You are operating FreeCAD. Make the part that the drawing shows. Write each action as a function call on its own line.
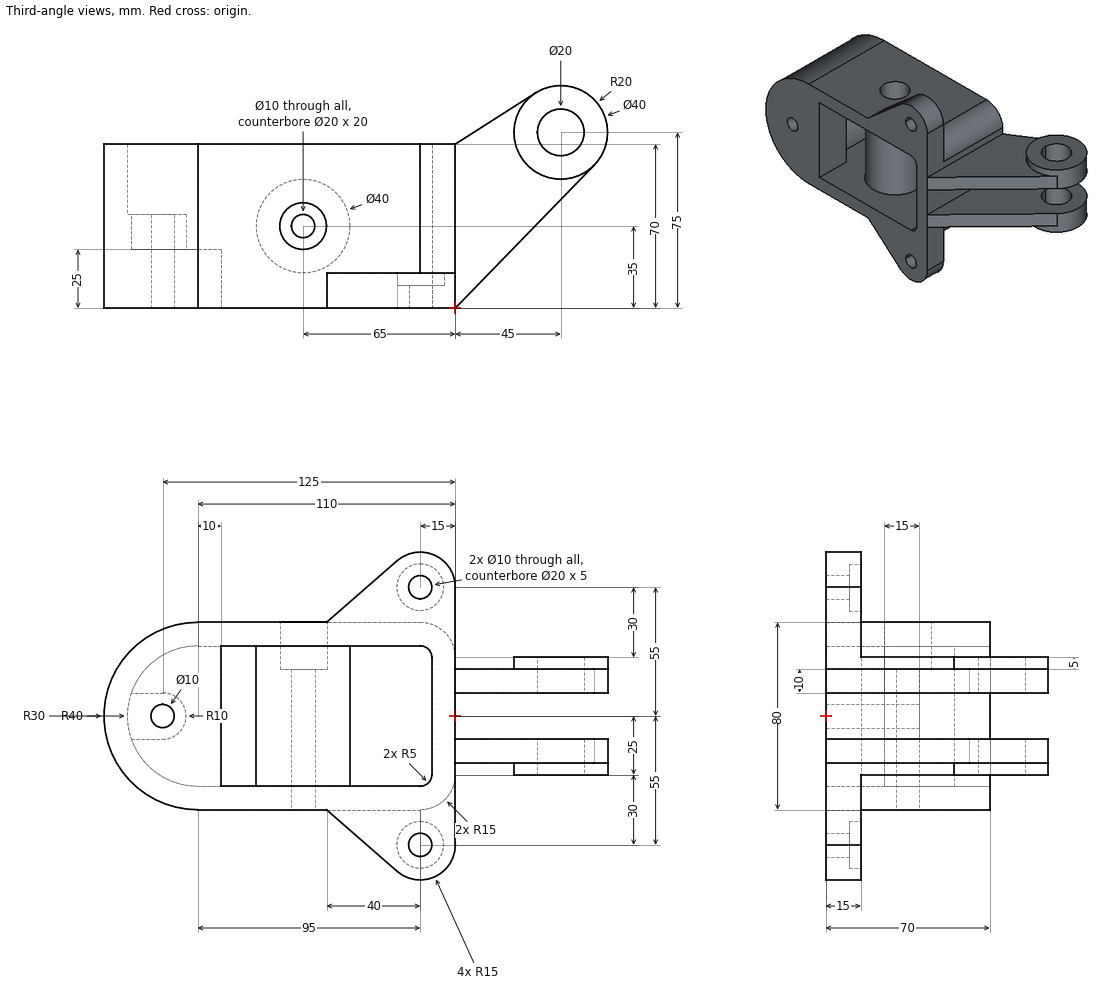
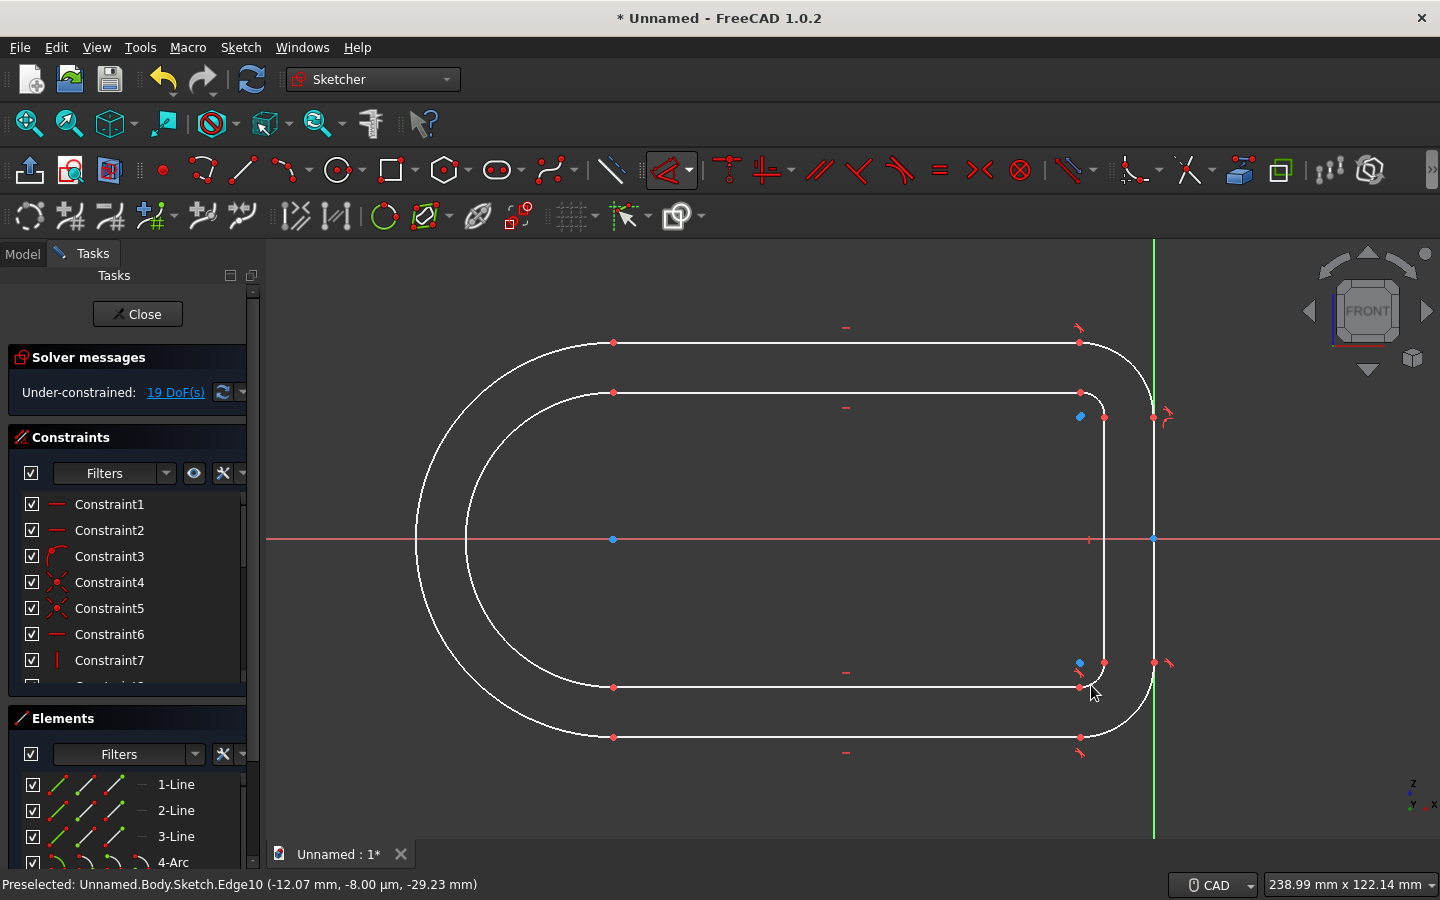
click(754, 687)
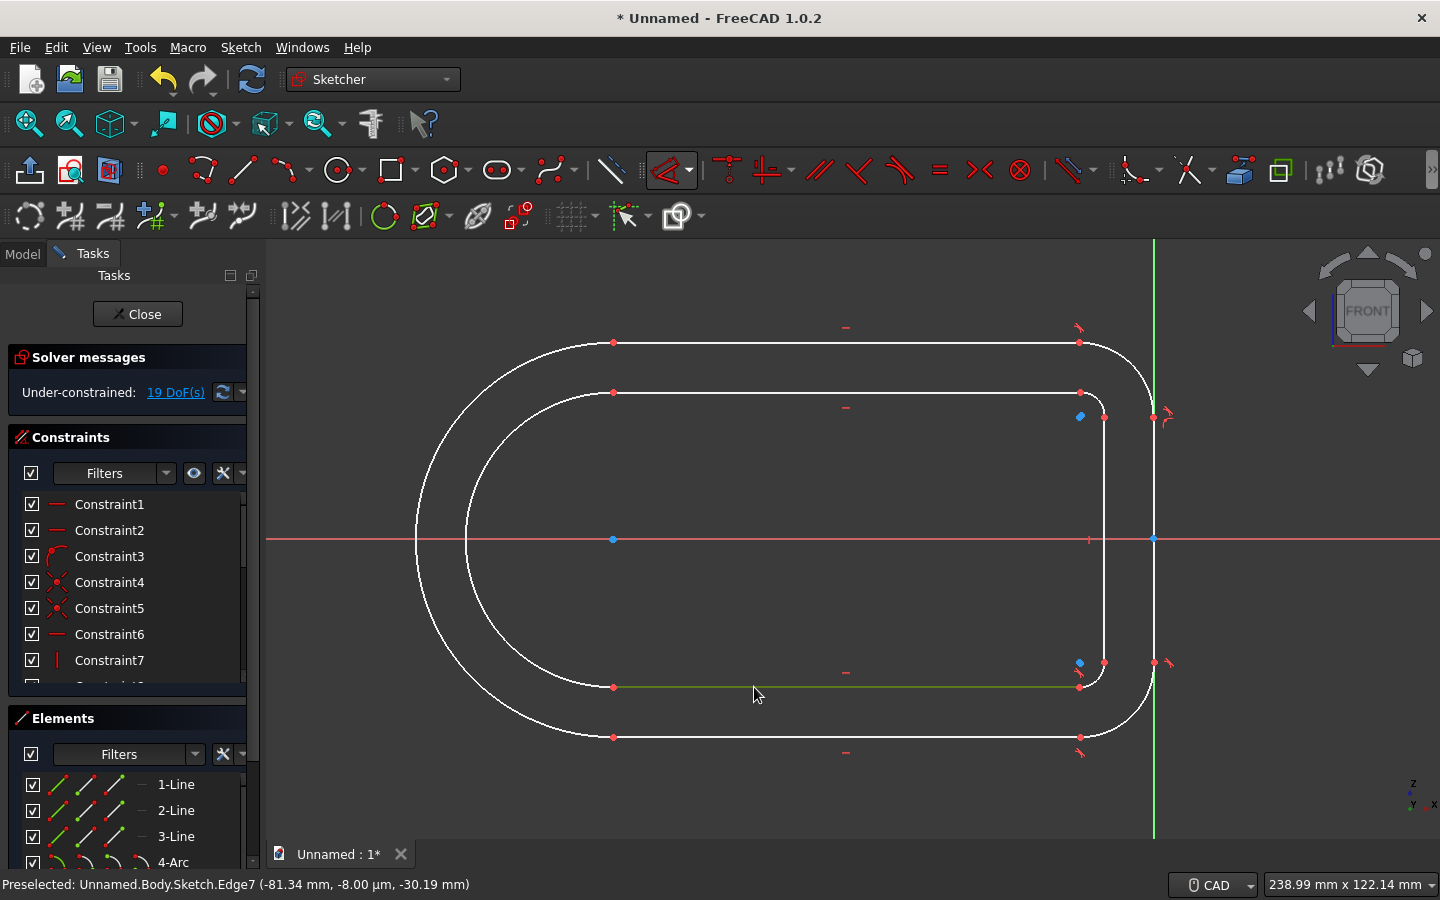
click(494, 453)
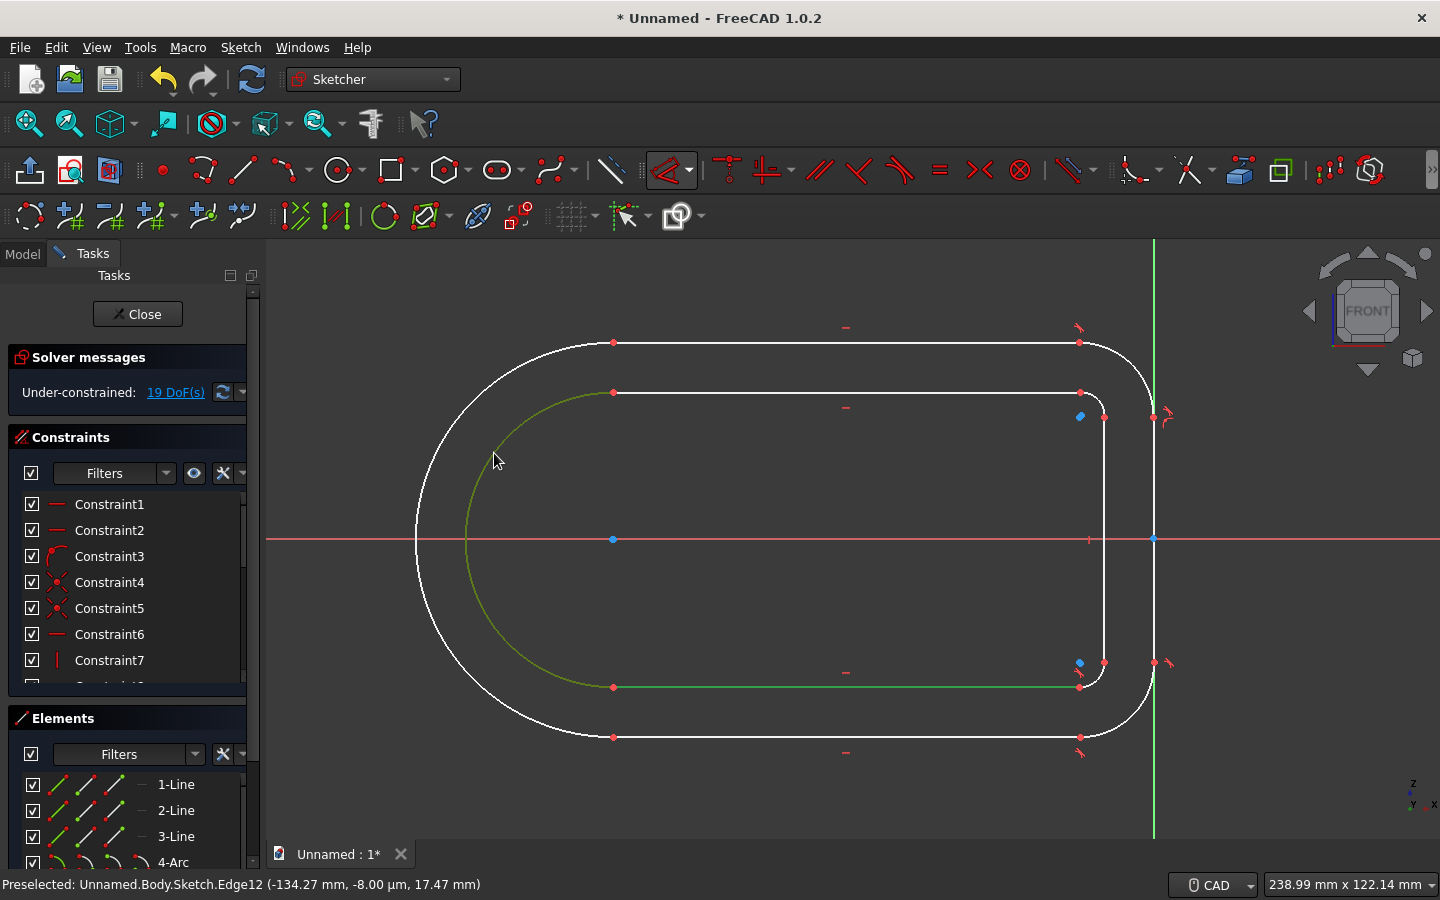
key(t)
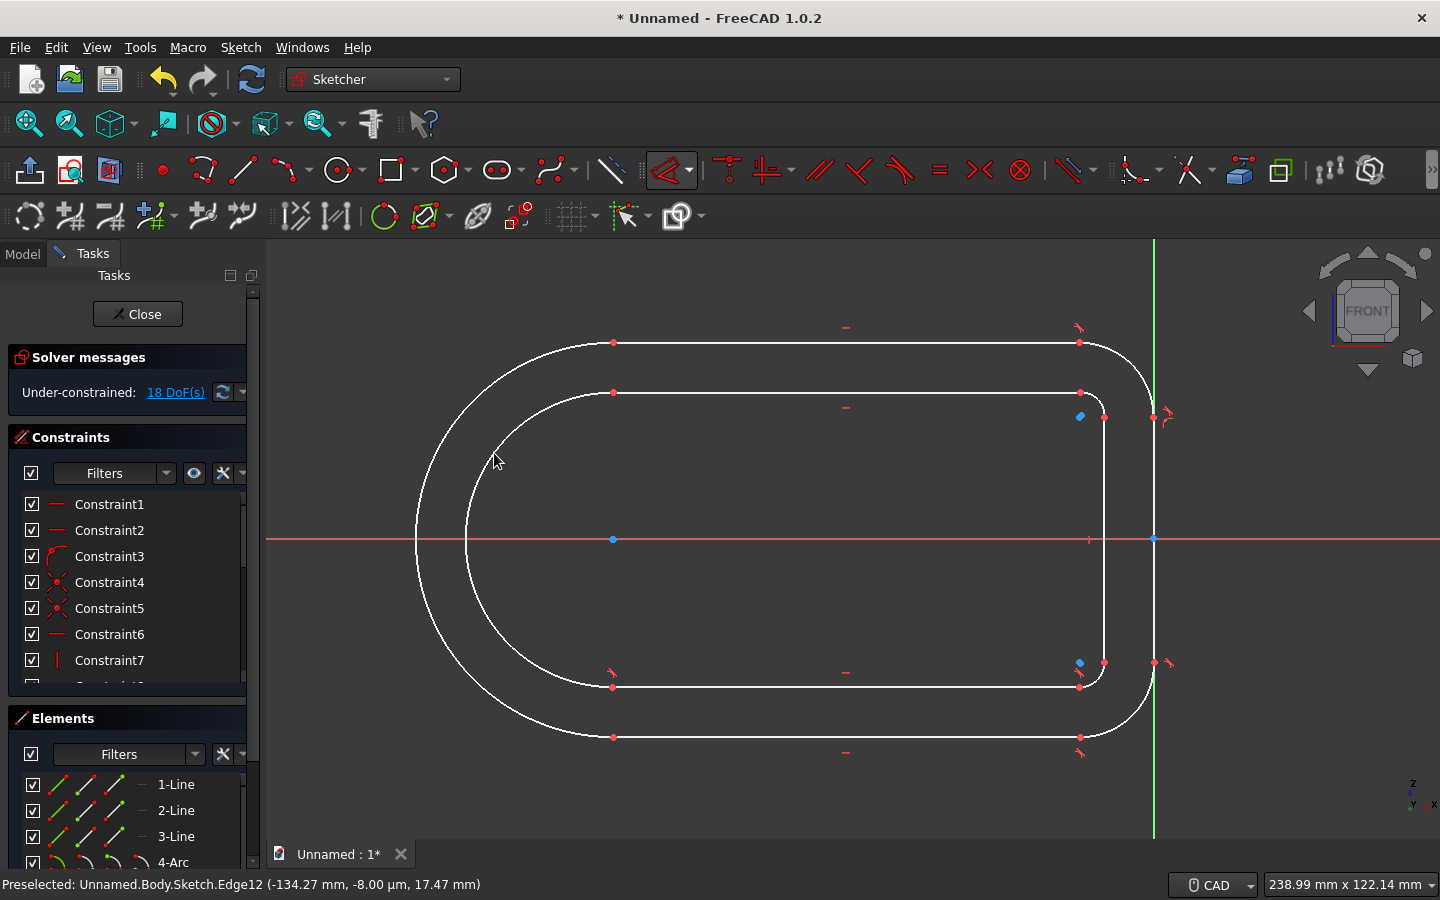
click(1104, 589)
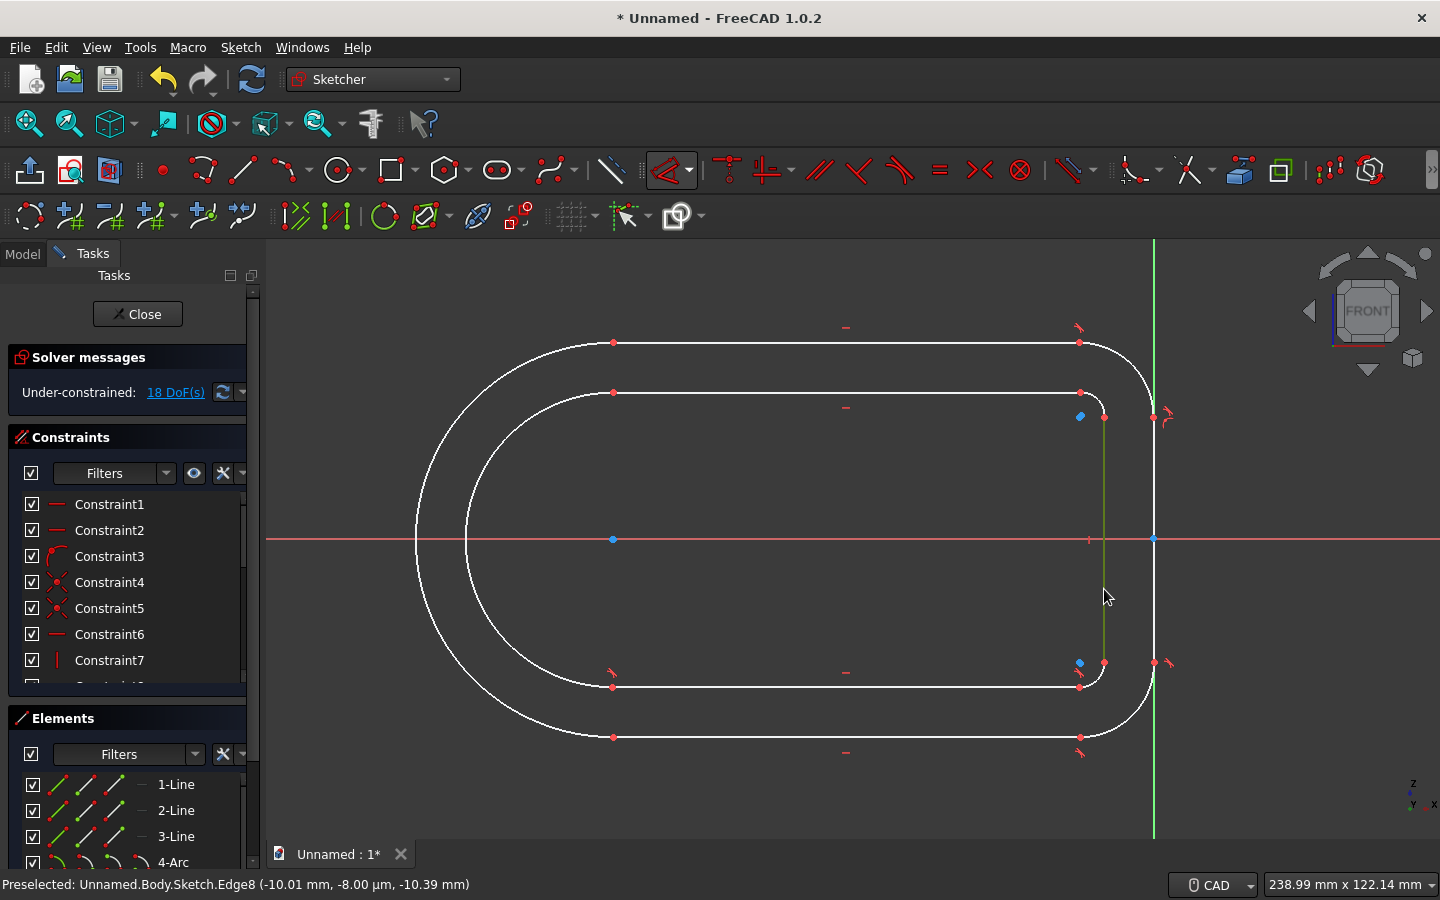
click(1091, 685)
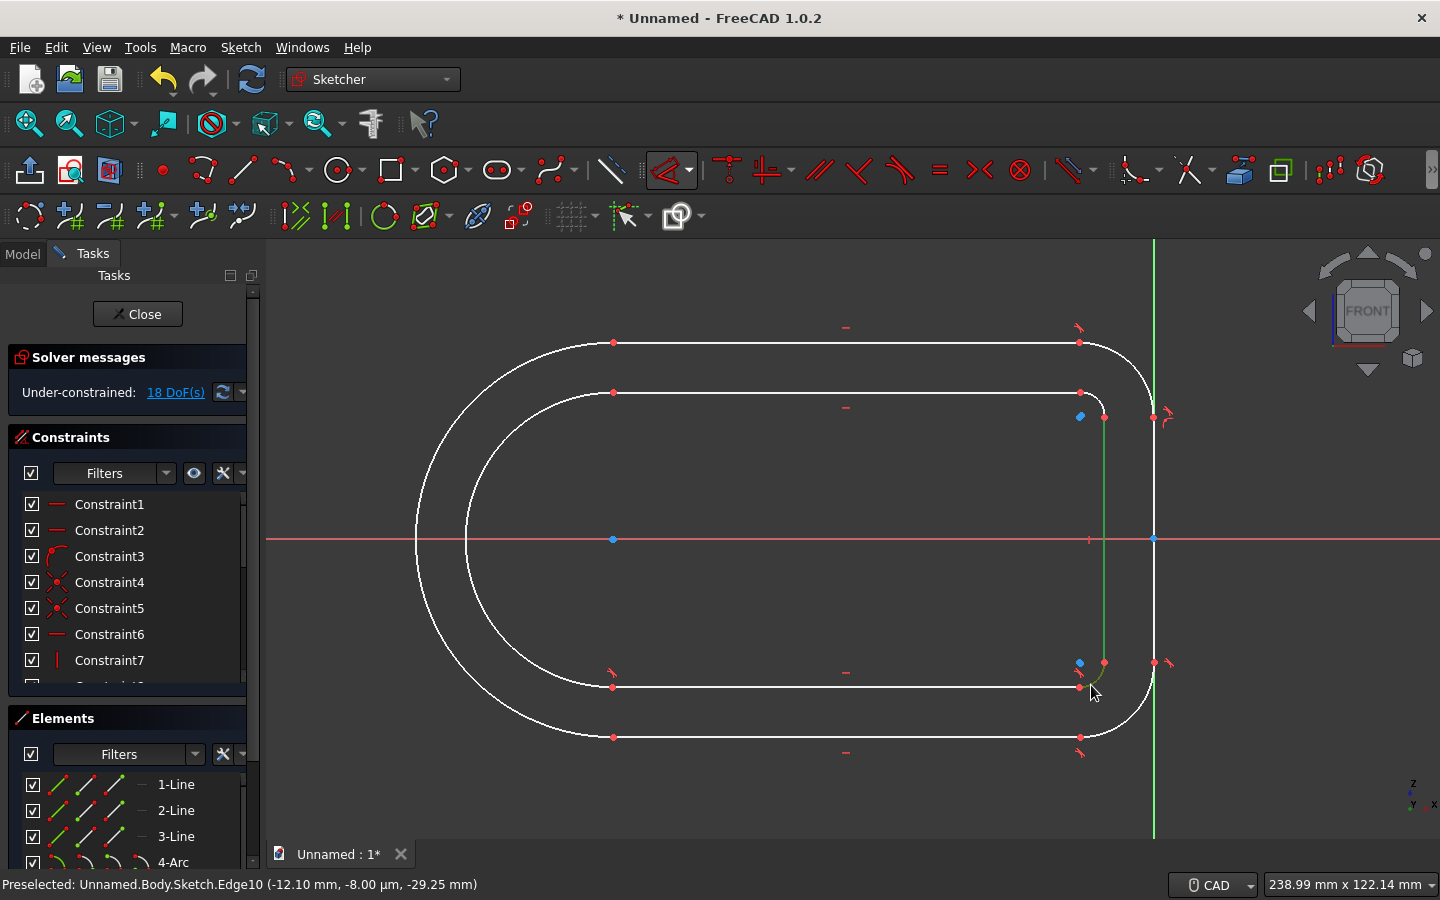
key(t)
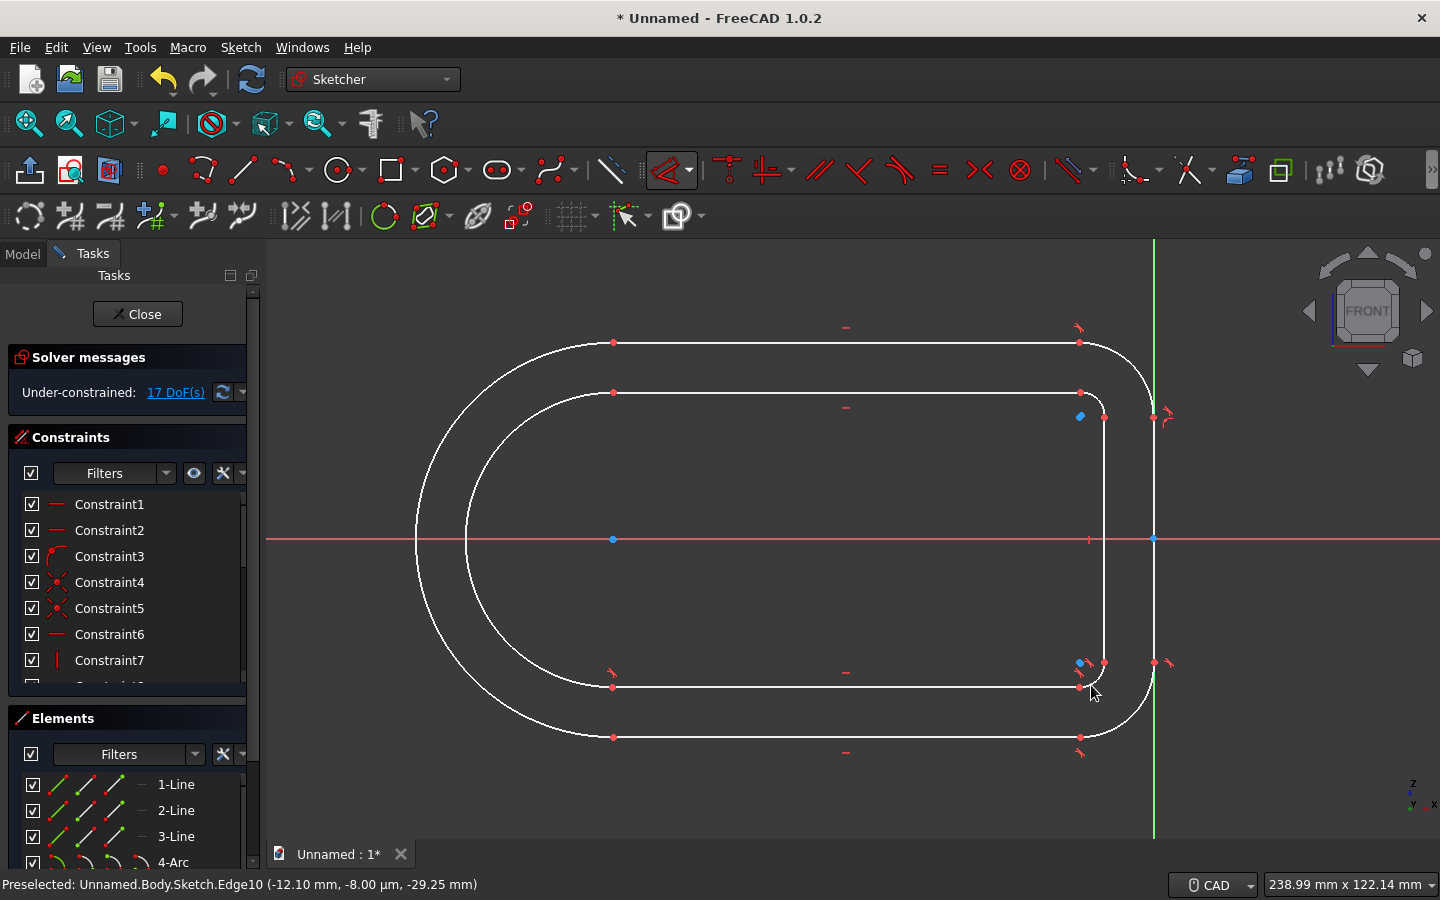
click(1104, 589)